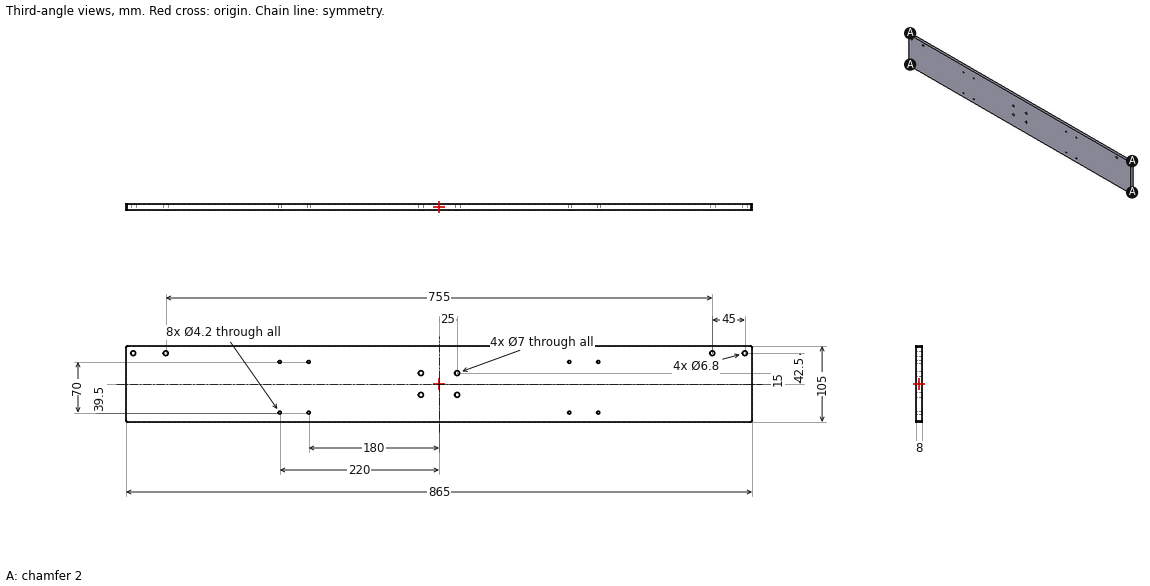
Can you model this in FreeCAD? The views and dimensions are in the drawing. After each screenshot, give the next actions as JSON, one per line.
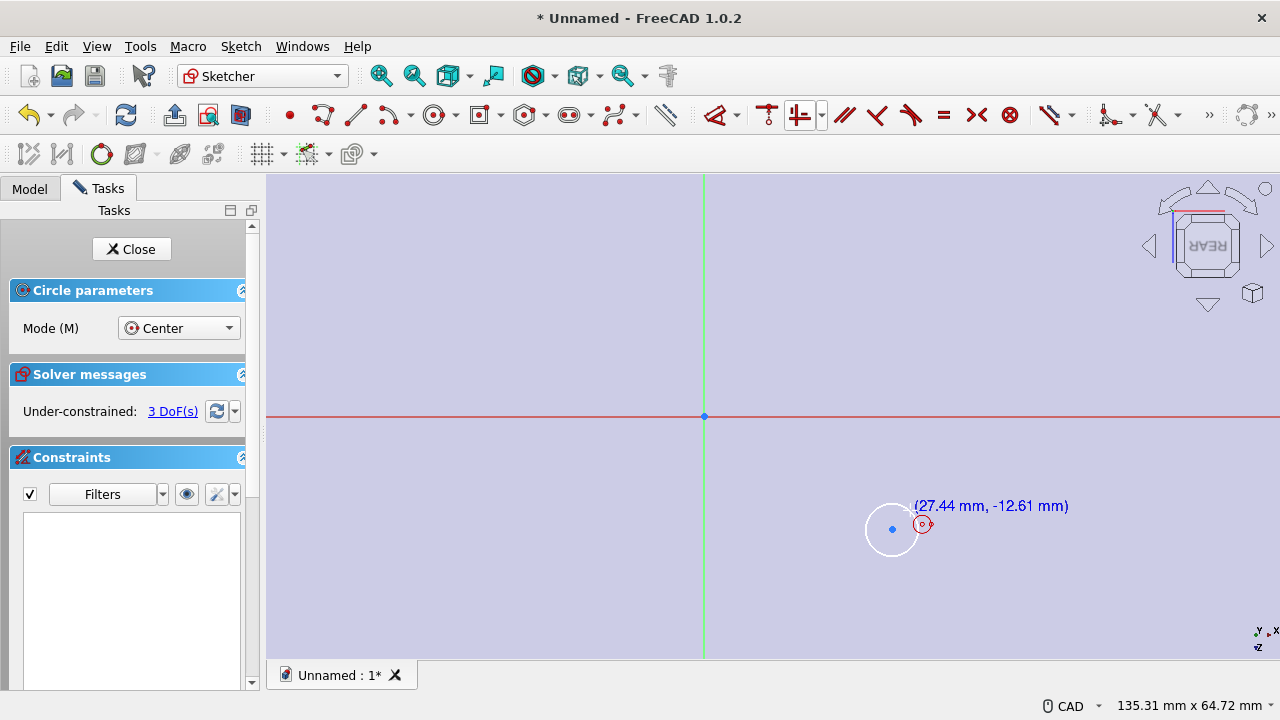
{"action": "left_click", "coordinate": [892, 304]}
{"action": "left_click", "coordinate": [910, 286]}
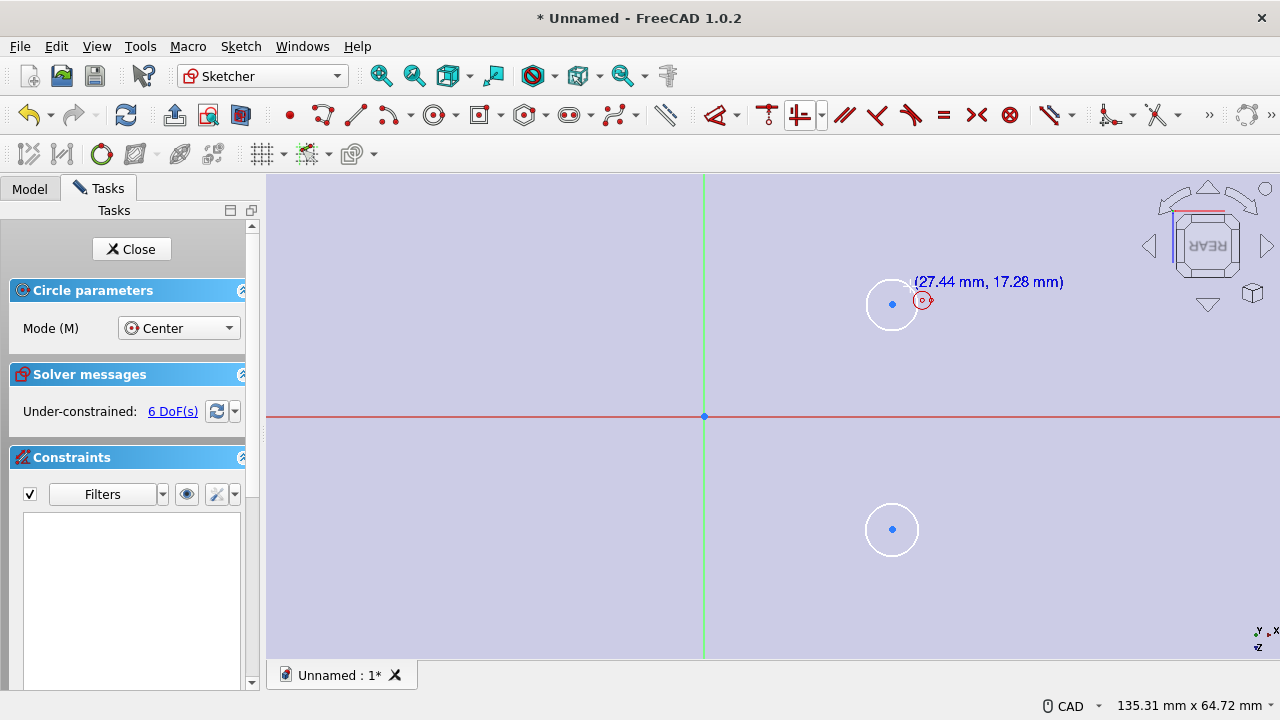
{"action": "left_click", "coordinate": [517, 304]}
{"action": "left_click", "coordinate": [536, 286]}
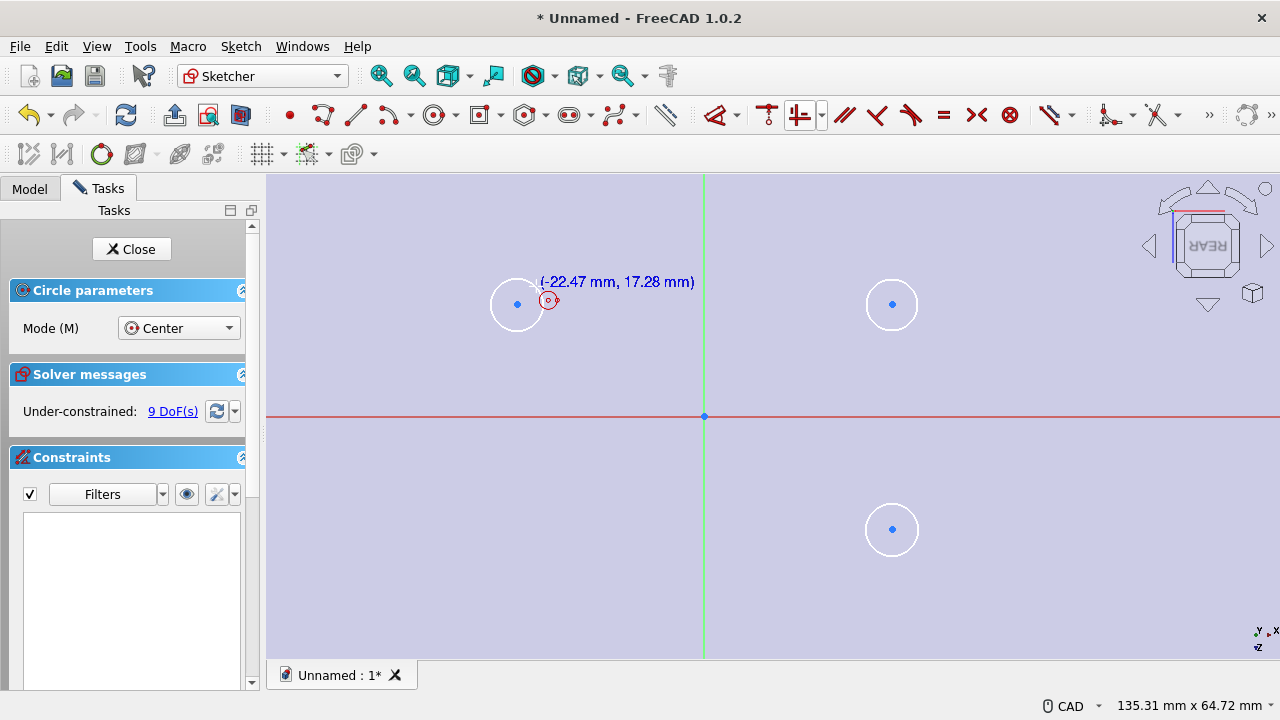
{"action": "left_click", "coordinate": [517, 529]}
{"action": "left_click", "coordinate": [536, 510]}
{"action": "key", "text": "Escape"}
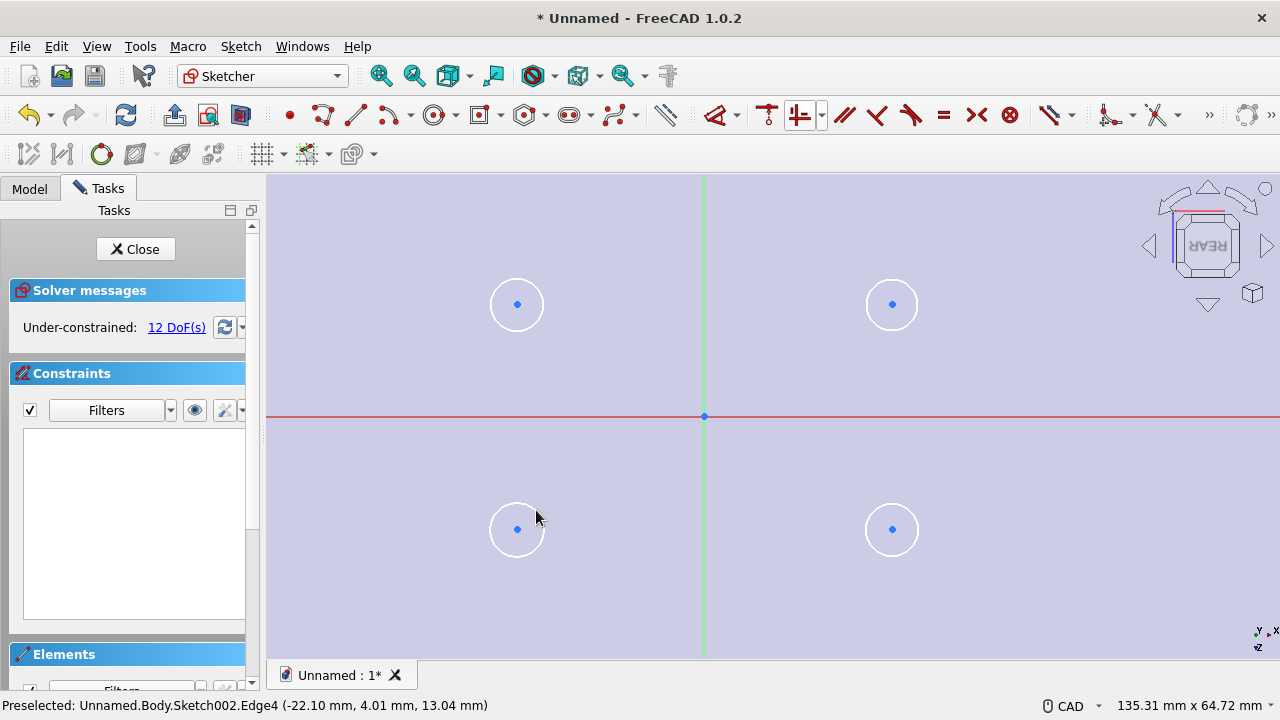
{"action": "left_click", "coordinate": [910, 511]}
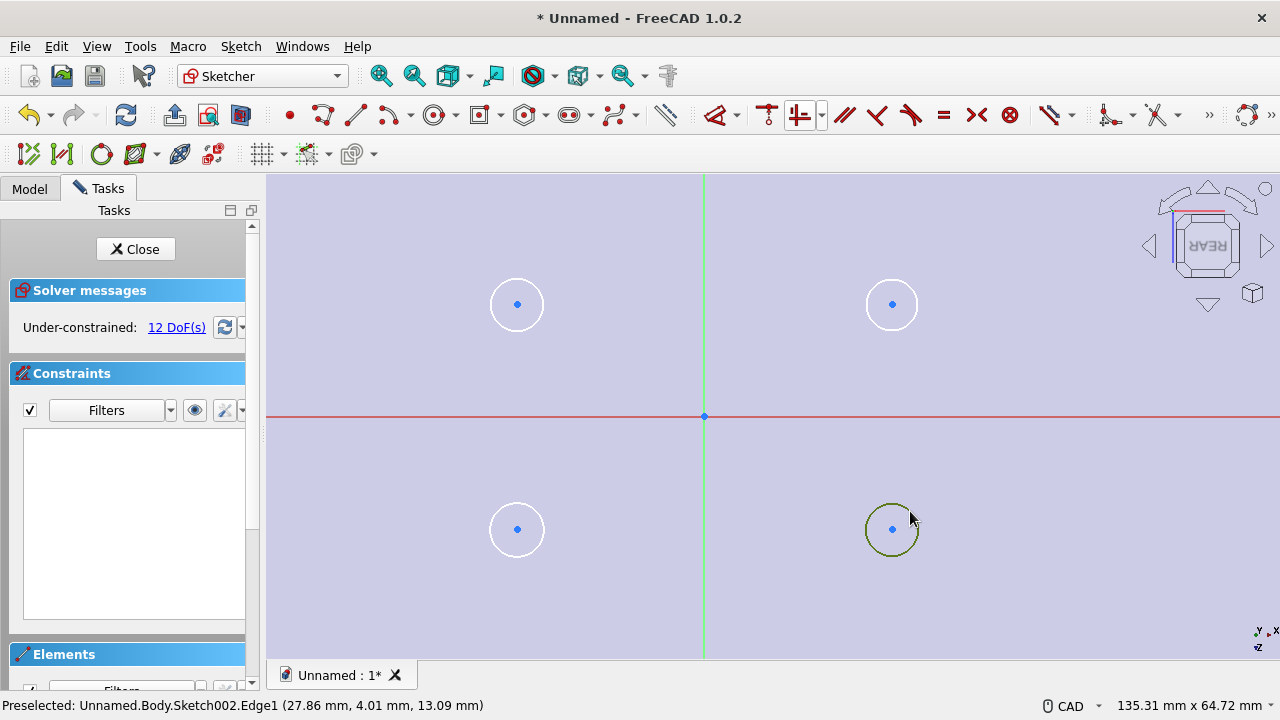
{"action": "left_click", "coordinate": [910, 287]}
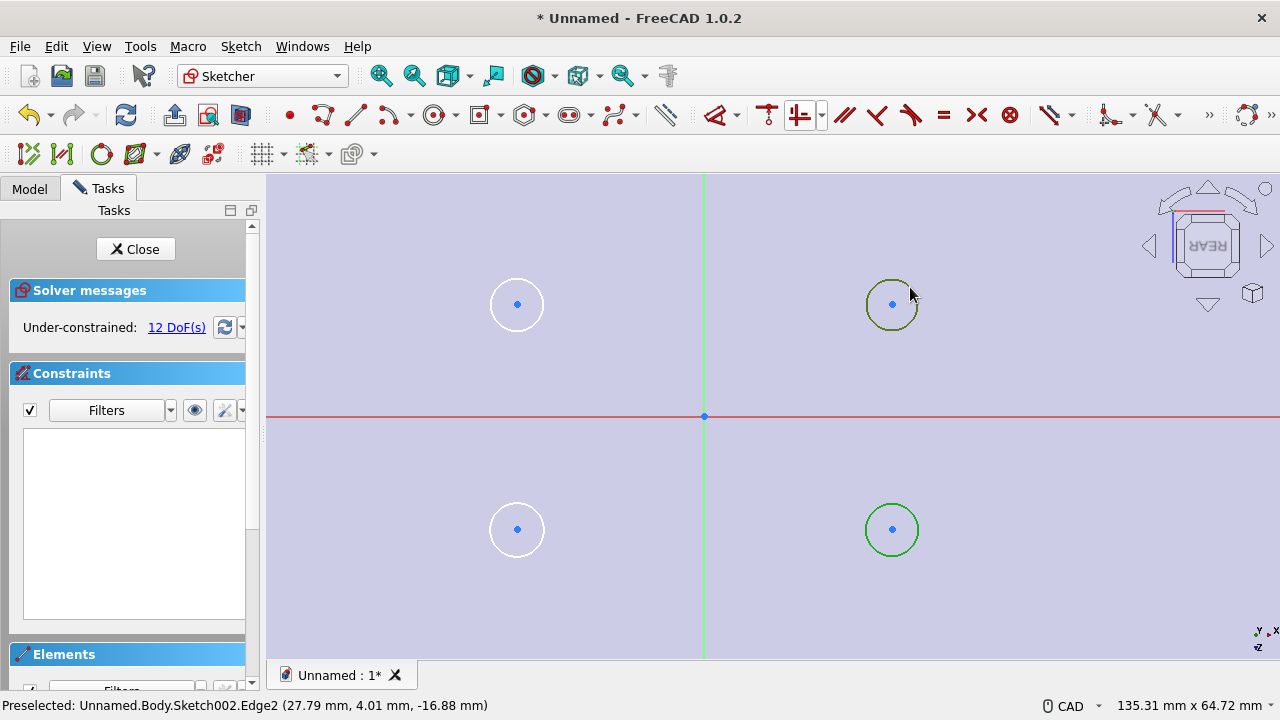
{"action": "left_click", "coordinate": [535, 286]}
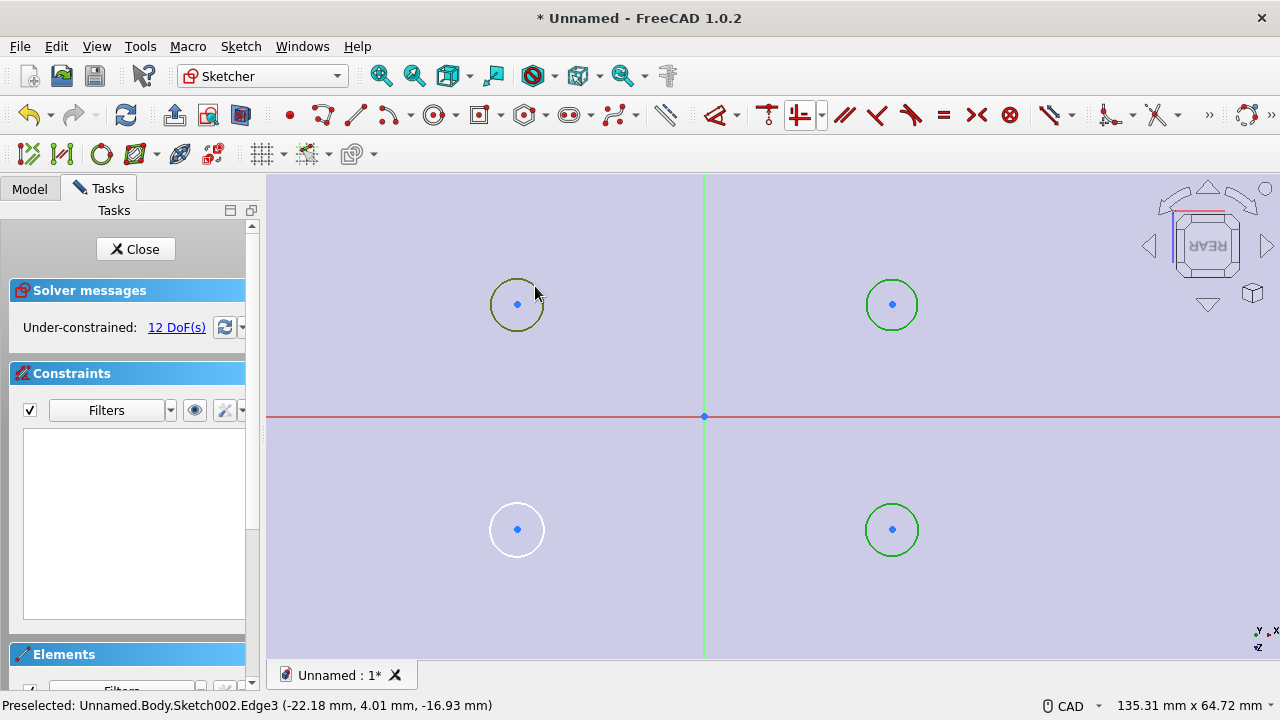
{"action": "left_click", "coordinate": [536, 511]}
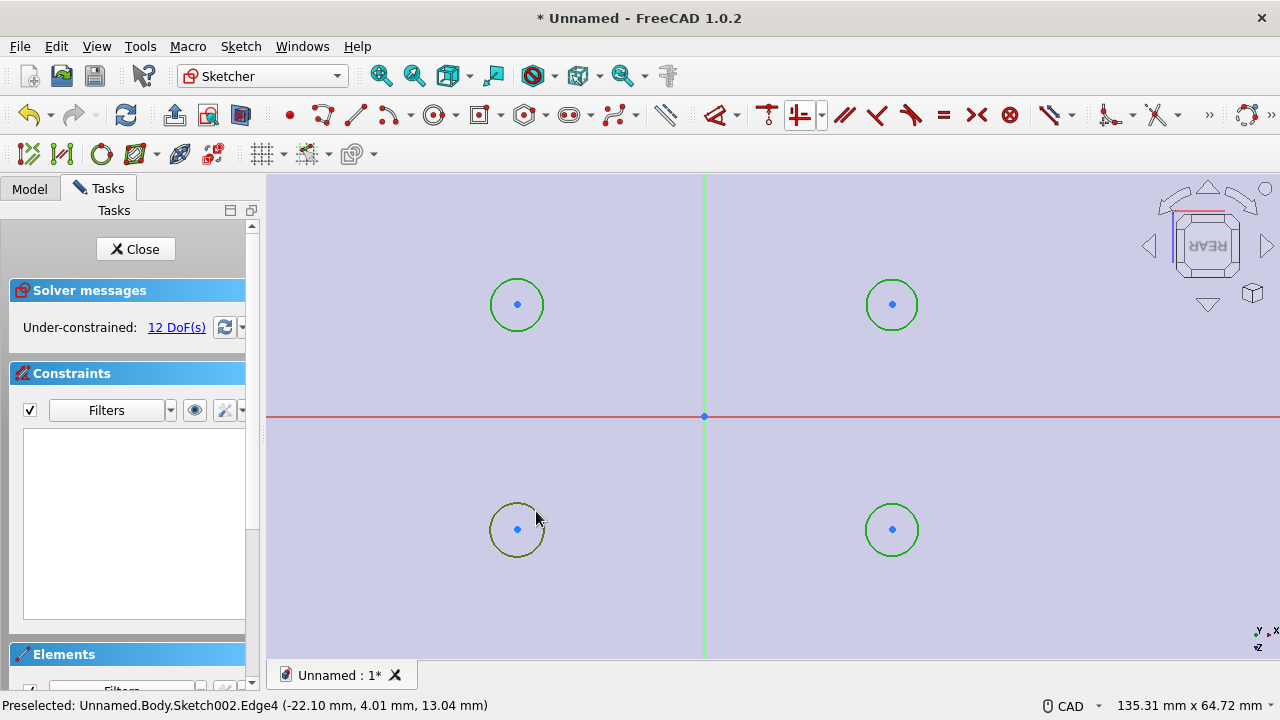
{"action": "key", "text": "e"}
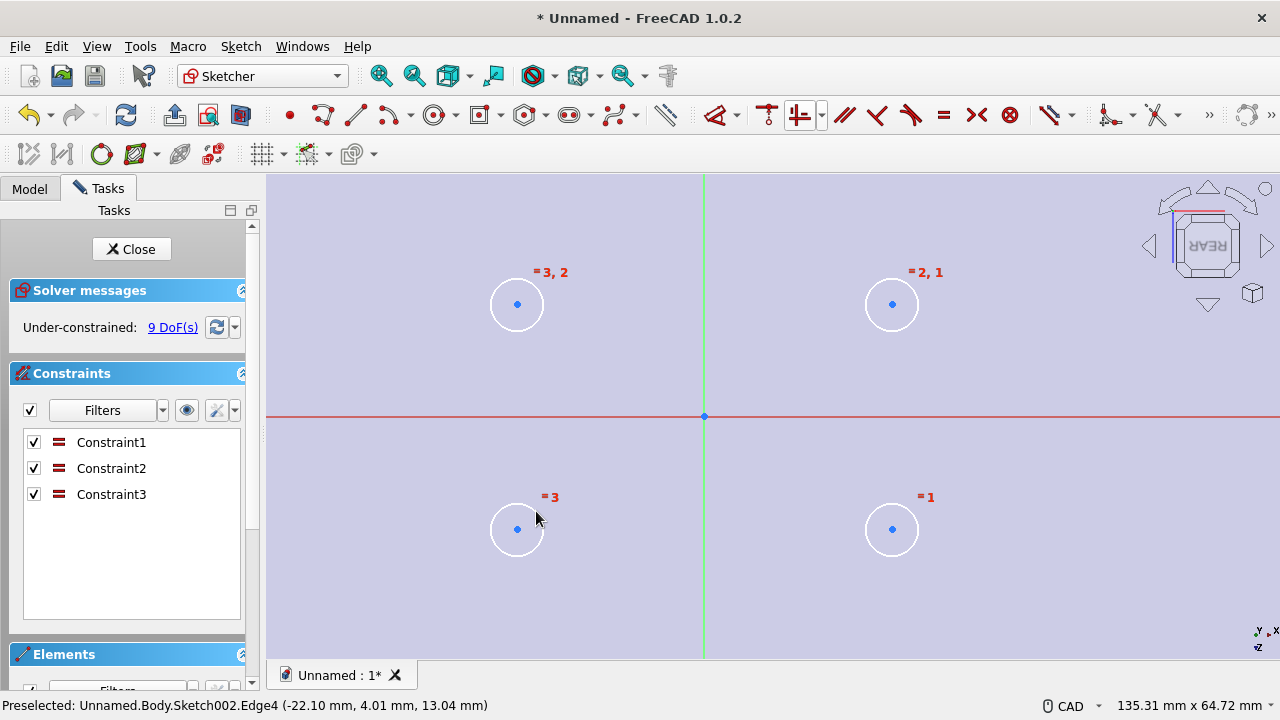
{"action": "left_click", "coordinate": [892, 530]}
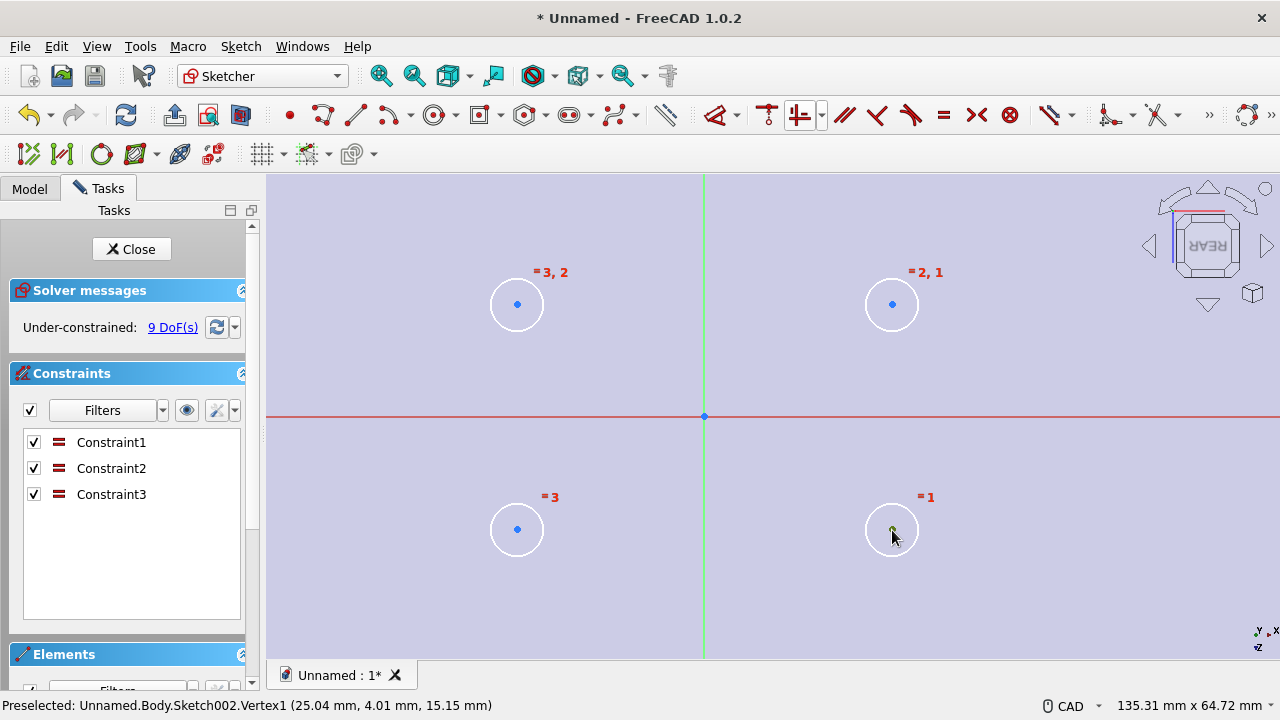
{"action": "left_click", "coordinate": [892, 305]}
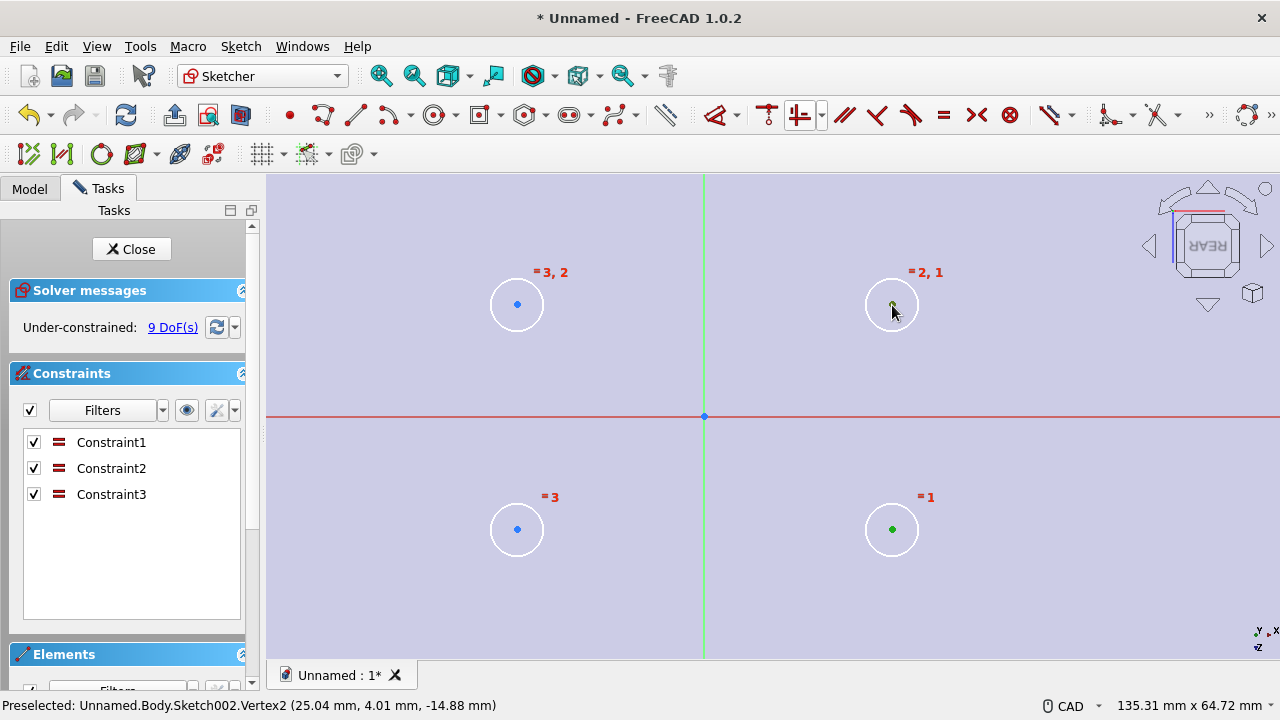
{"action": "left_click", "coordinate": [353, 416]}